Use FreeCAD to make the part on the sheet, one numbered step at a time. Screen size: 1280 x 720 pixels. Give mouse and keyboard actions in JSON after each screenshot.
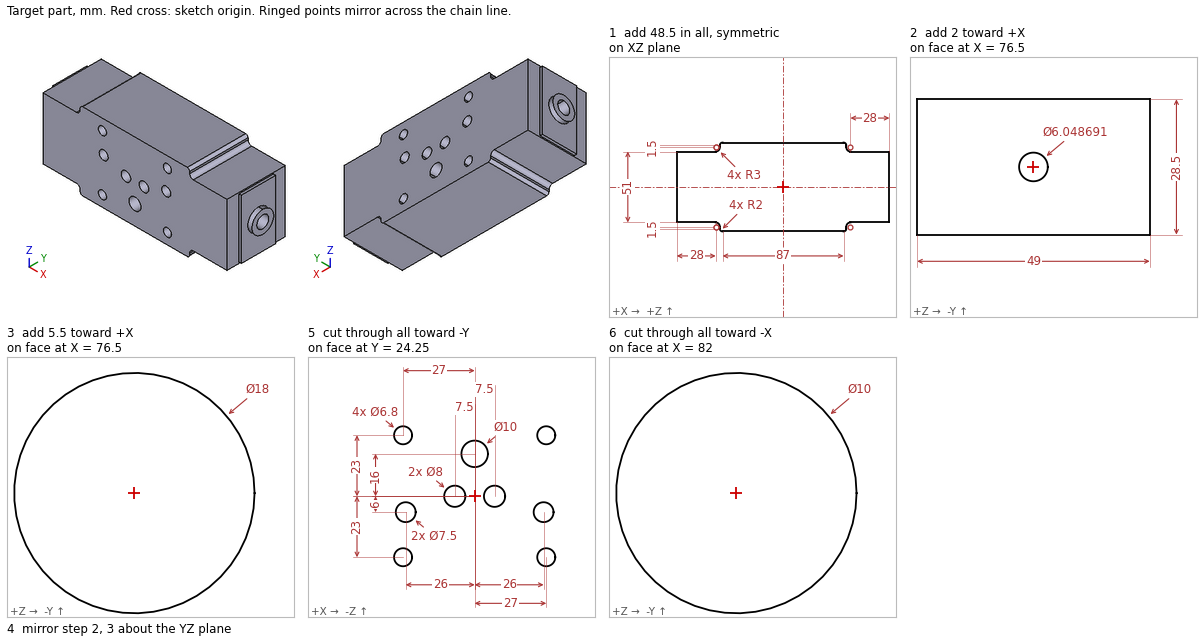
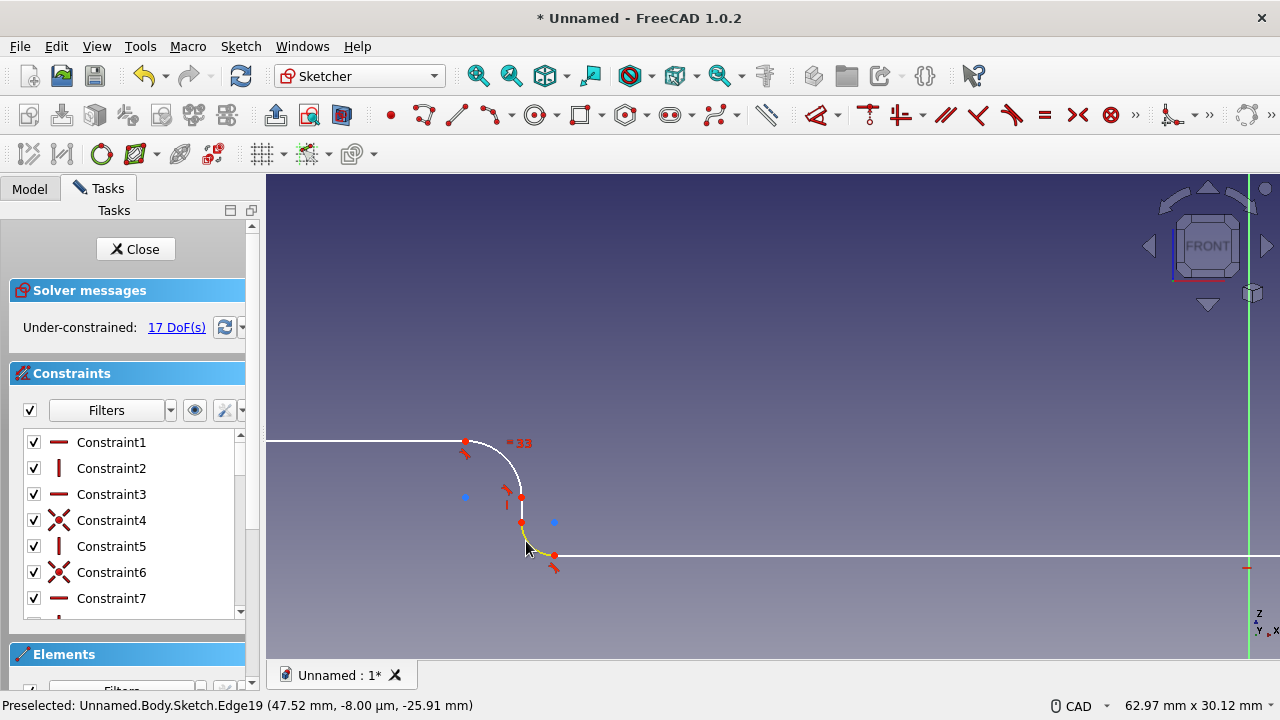
{"action": "left_click", "coordinate": [525, 538]}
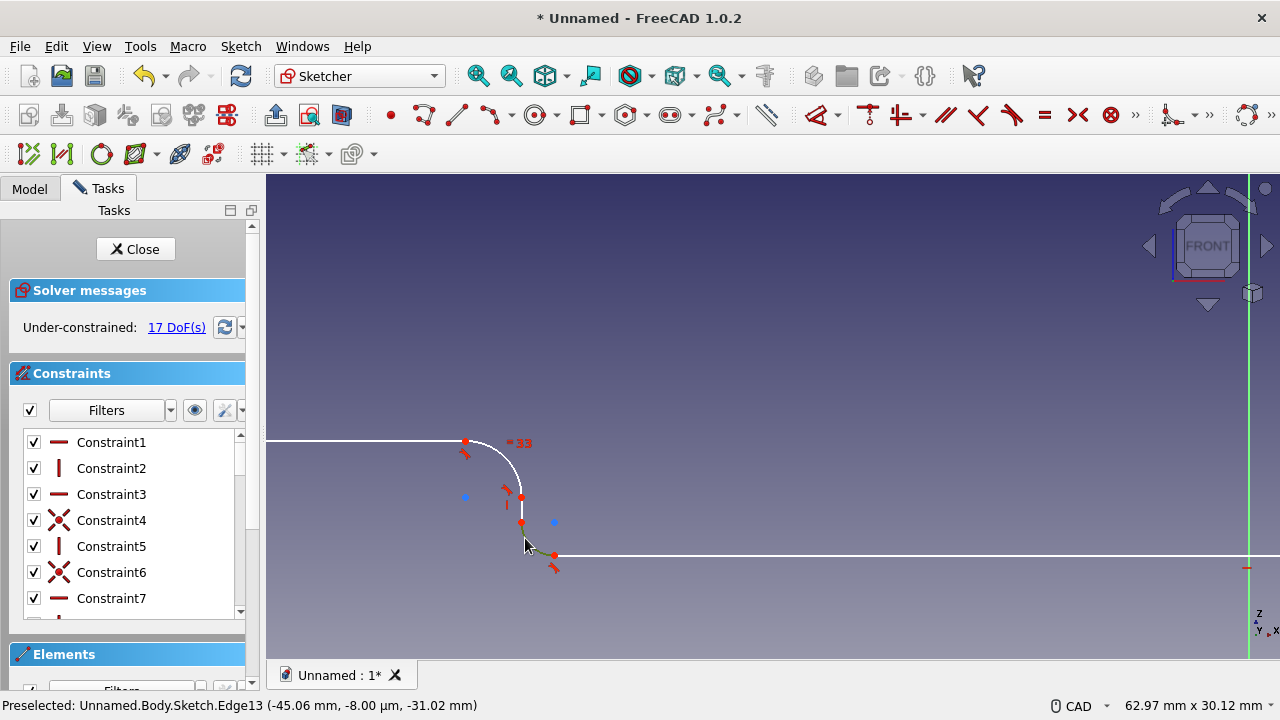
{"action": "scroll", "coordinate": [526, 541], "scroll_direction": "down", "scroll_amount": 7}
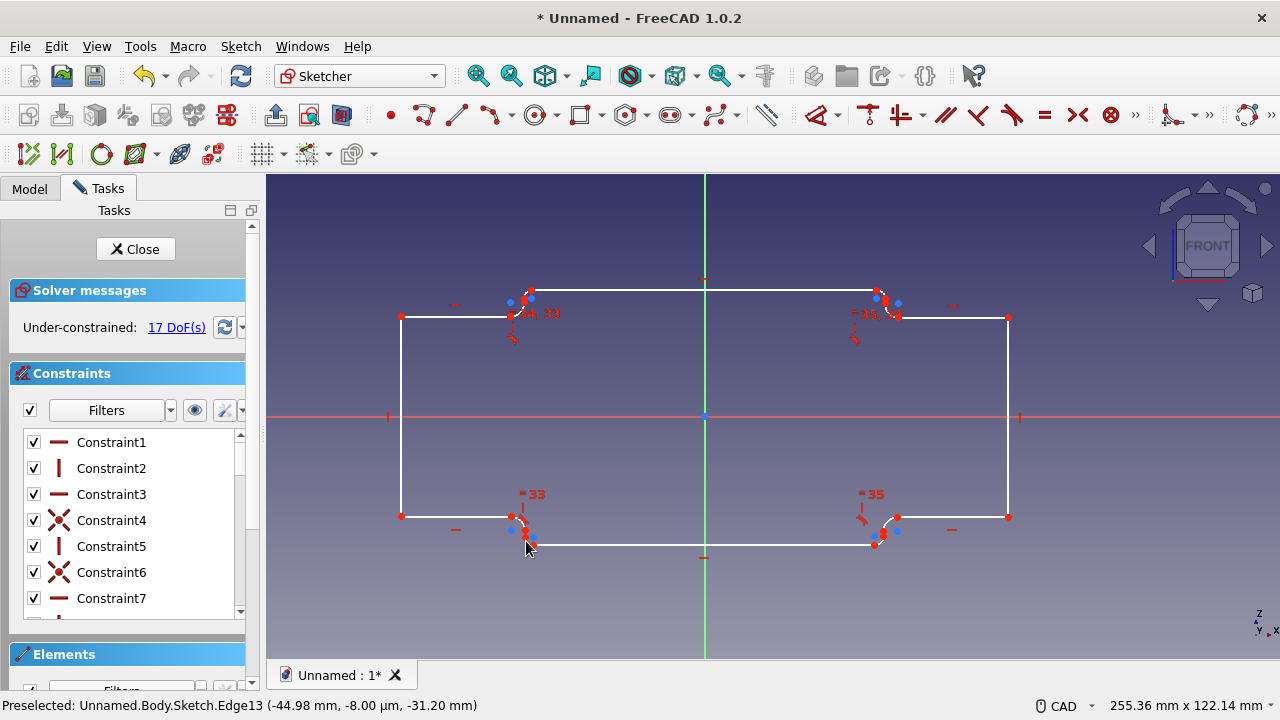
{"action": "scroll", "coordinate": [528, 291], "scroll_direction": "up", "scroll_amount": 7}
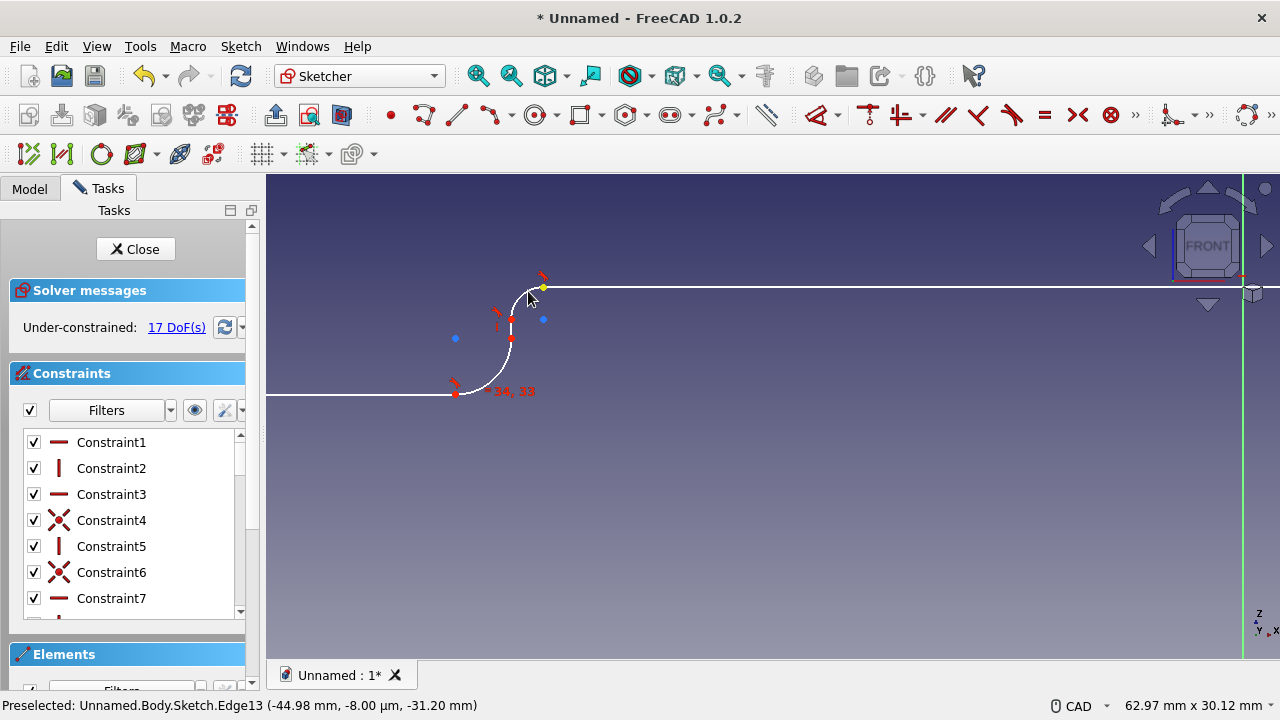
{"action": "left_click", "coordinate": [529, 291]}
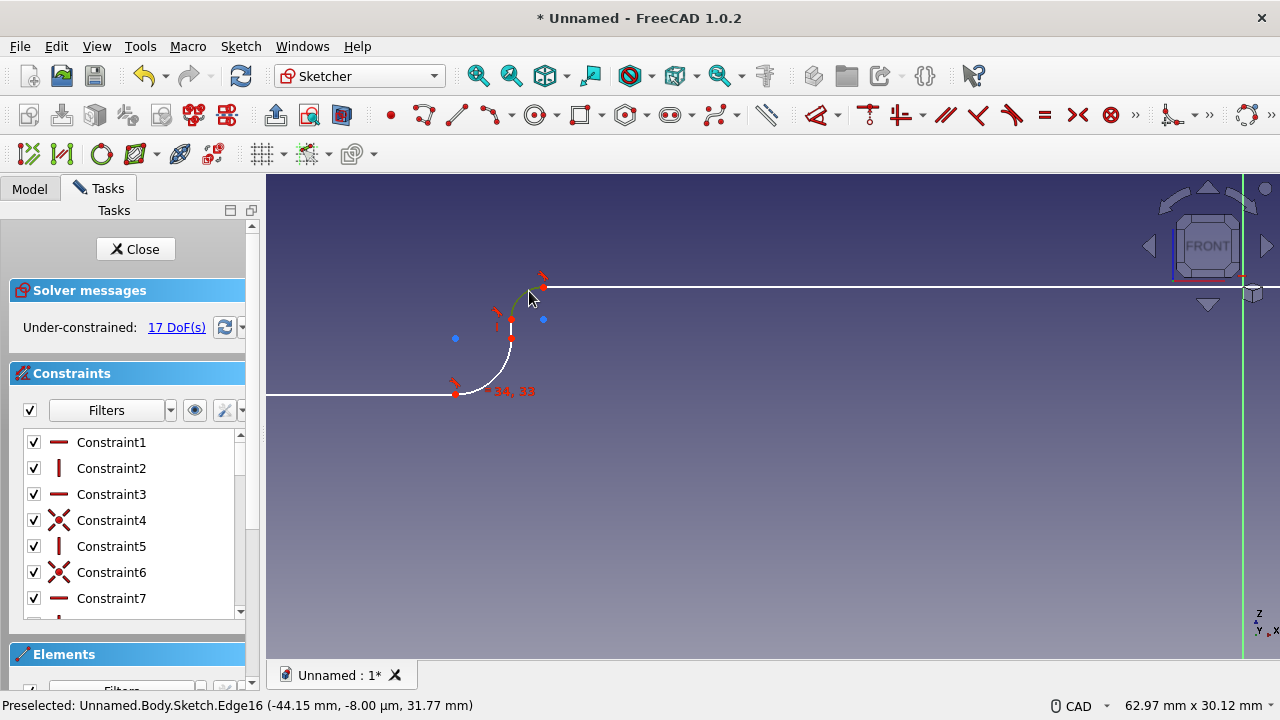
{"action": "scroll", "coordinate": [528, 291], "scroll_direction": "down", "scroll_amount": 7}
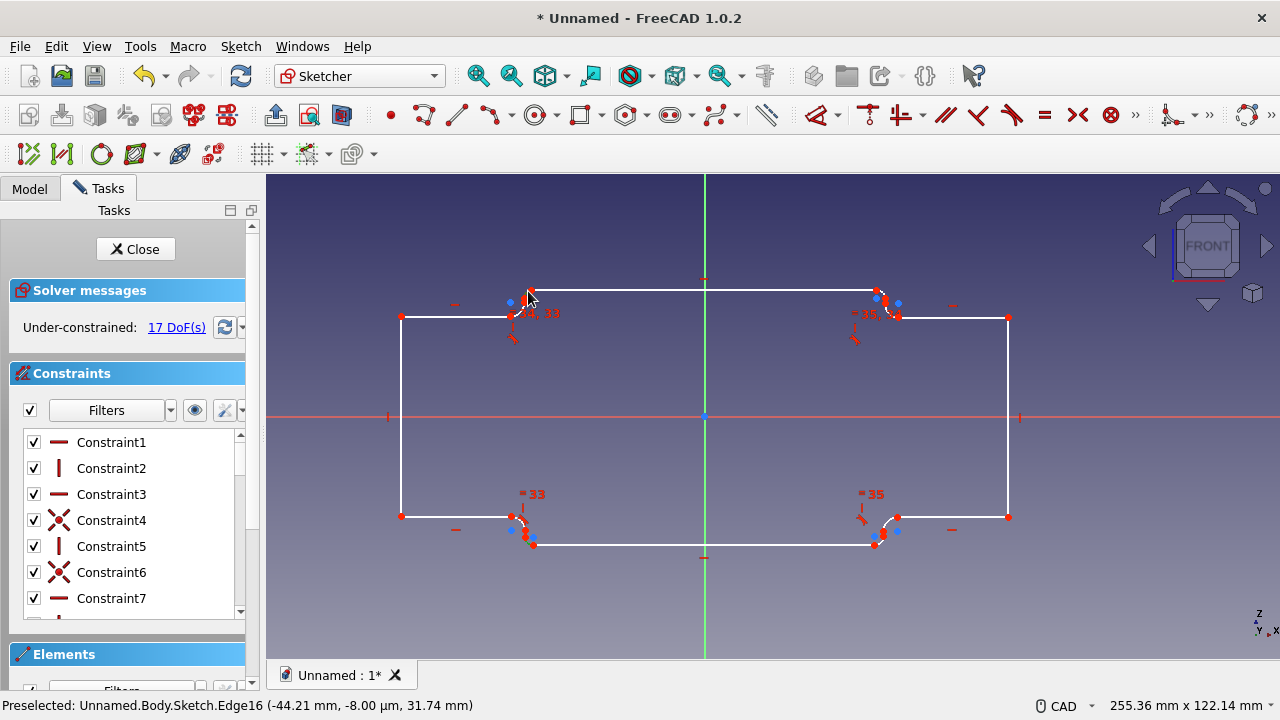
{"action": "scroll", "coordinate": [884, 295], "scroll_direction": "up", "scroll_amount": 7}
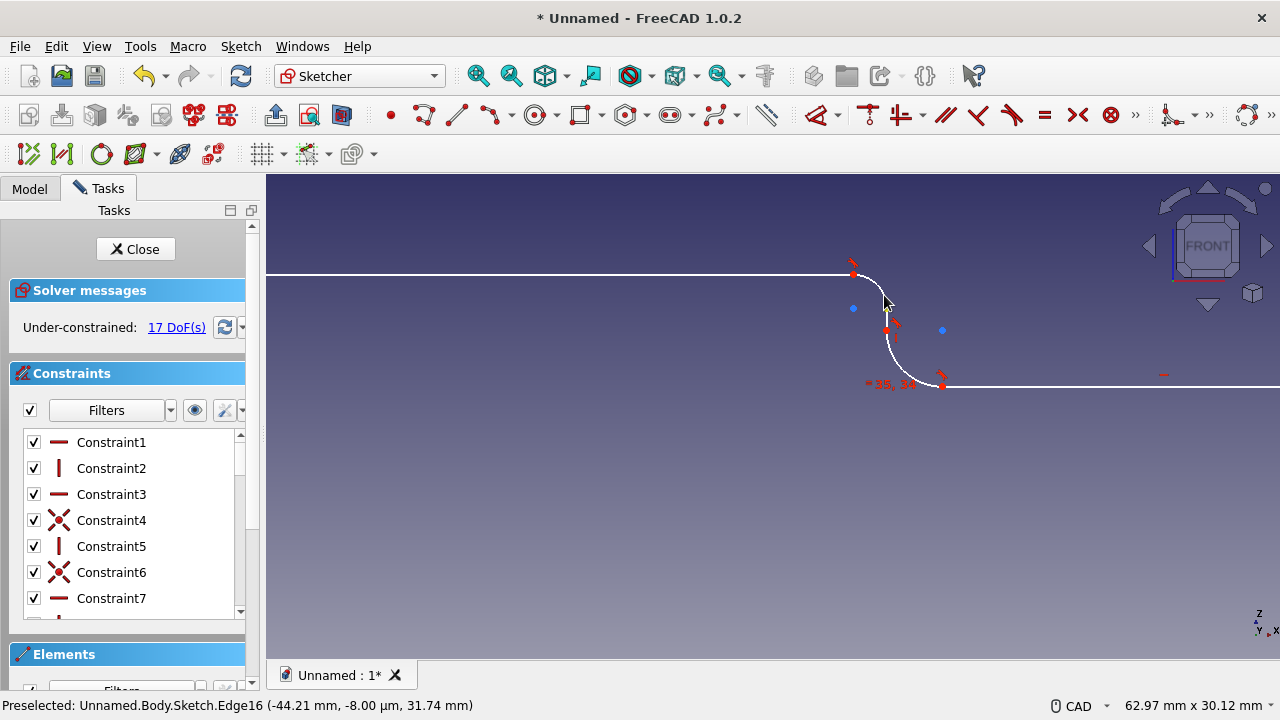
{"action": "left_click", "coordinate": [883, 293]}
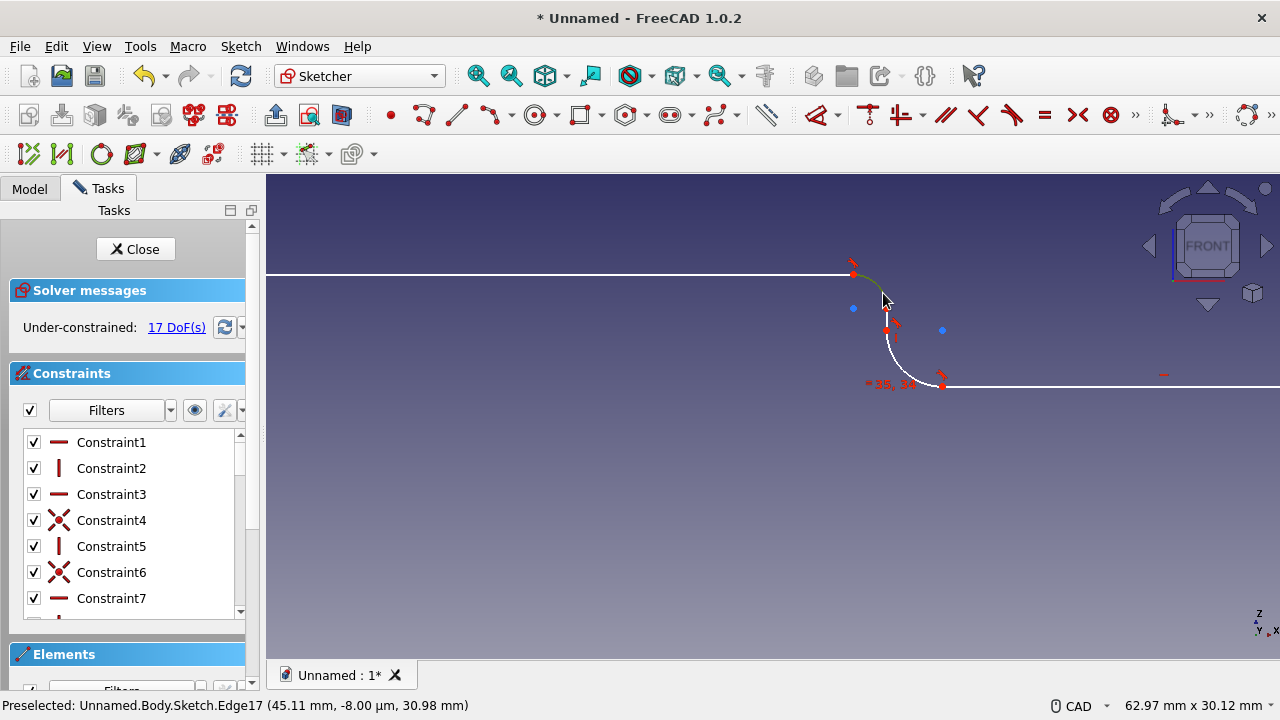
{"action": "scroll", "coordinate": [884, 295], "scroll_direction": "down", "scroll_amount": 7}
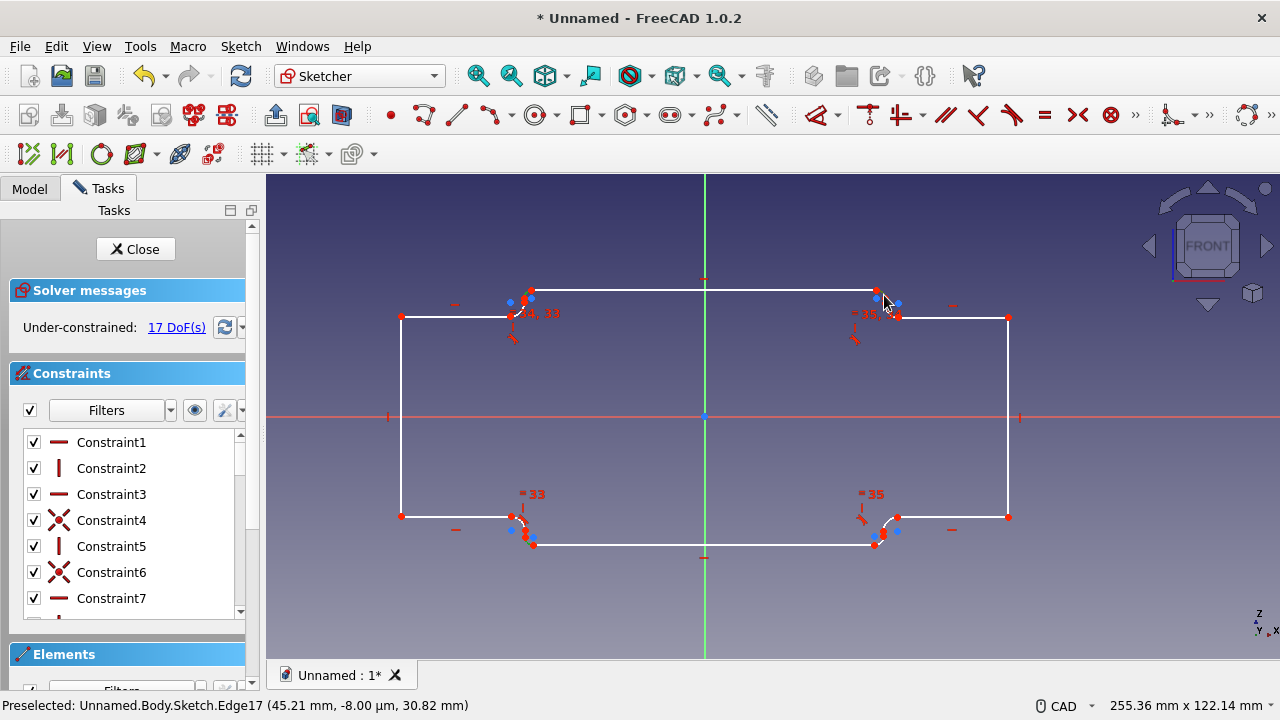
{"action": "scroll", "coordinate": [879, 544], "scroll_direction": "up", "scroll_amount": 7}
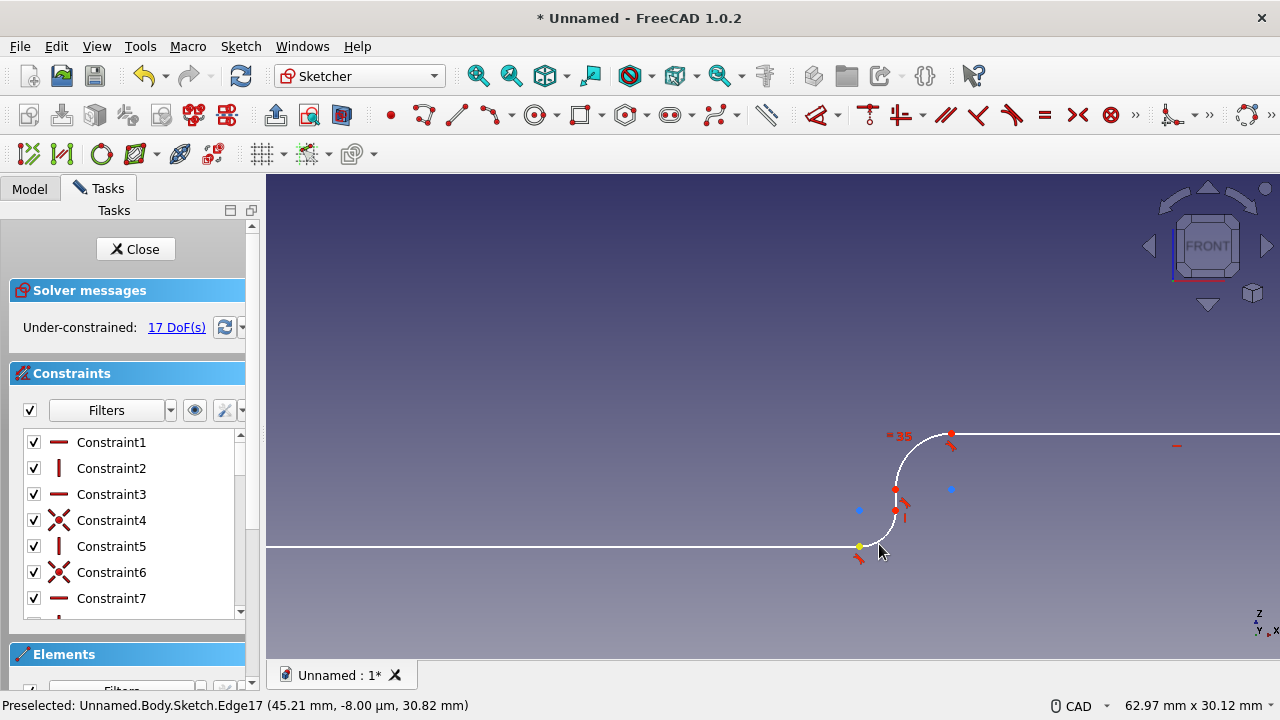
{"action": "left_click", "coordinate": [876, 543]}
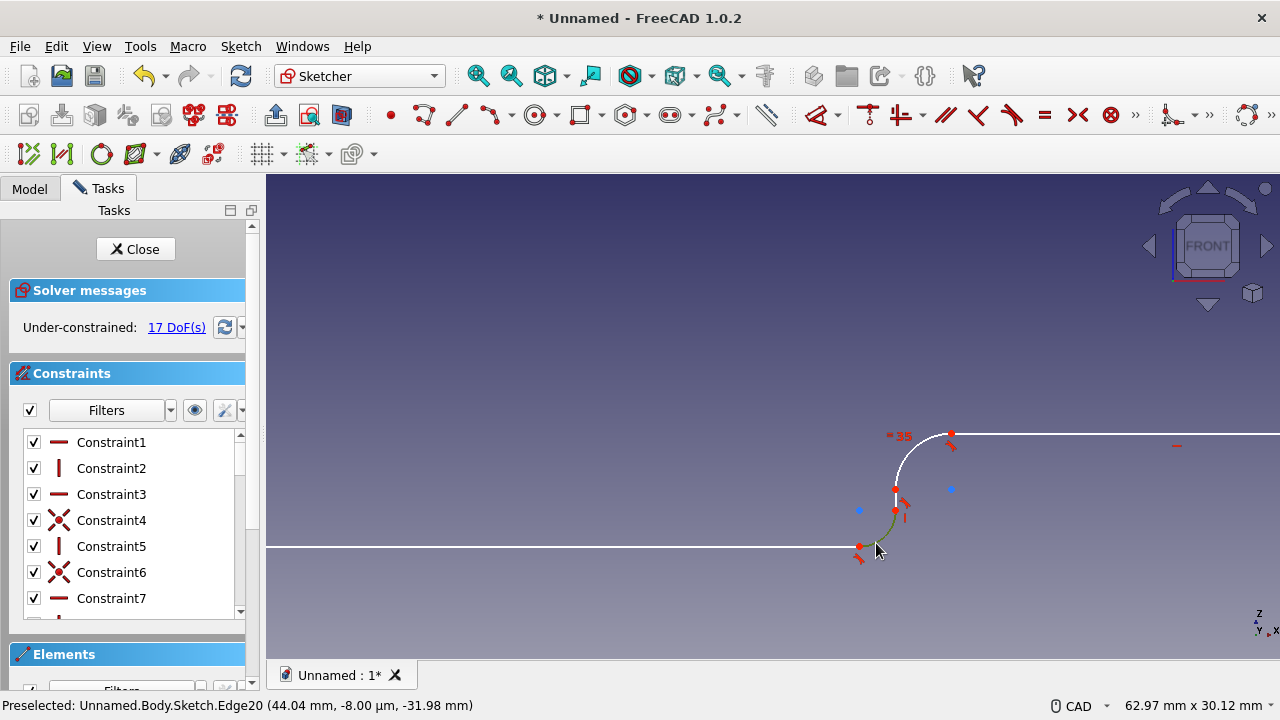
{"action": "key", "text": "e"}